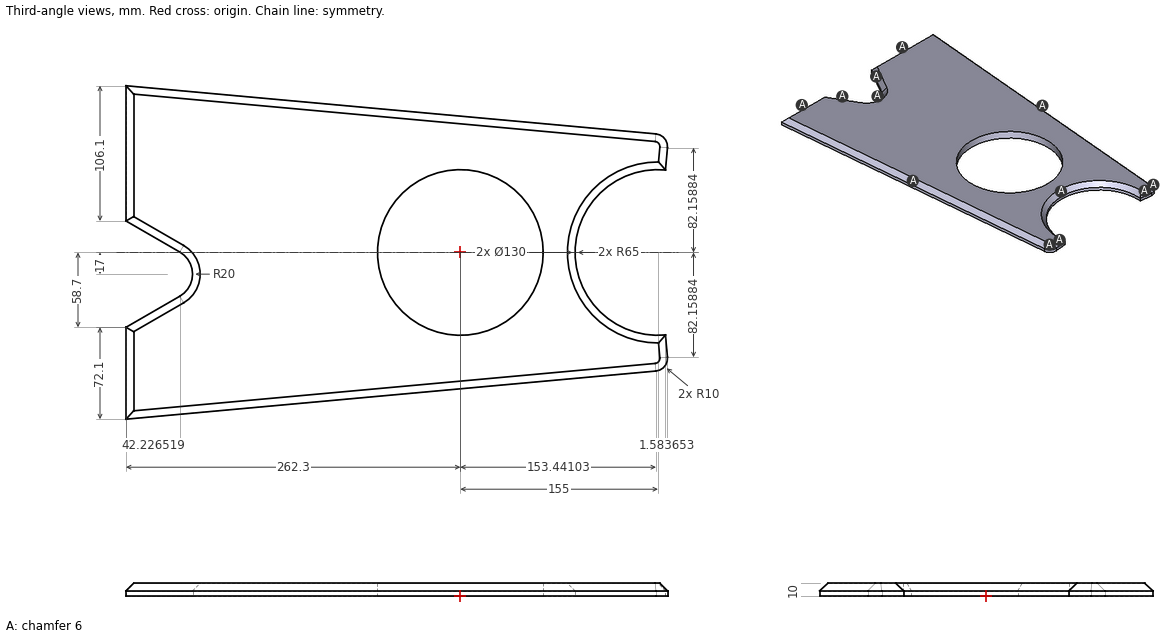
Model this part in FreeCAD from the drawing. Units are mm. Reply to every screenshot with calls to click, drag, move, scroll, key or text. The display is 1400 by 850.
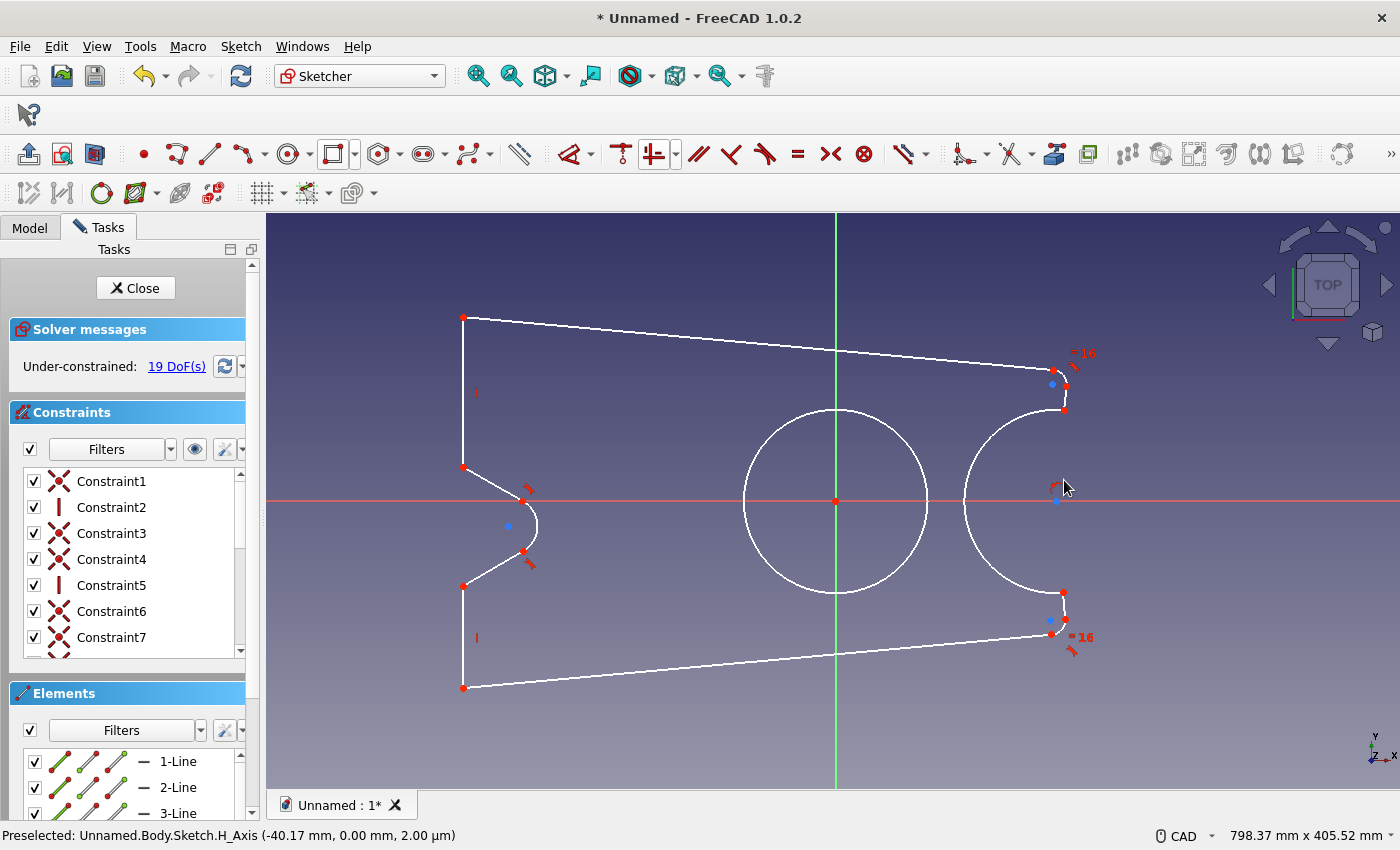
click(1051, 620)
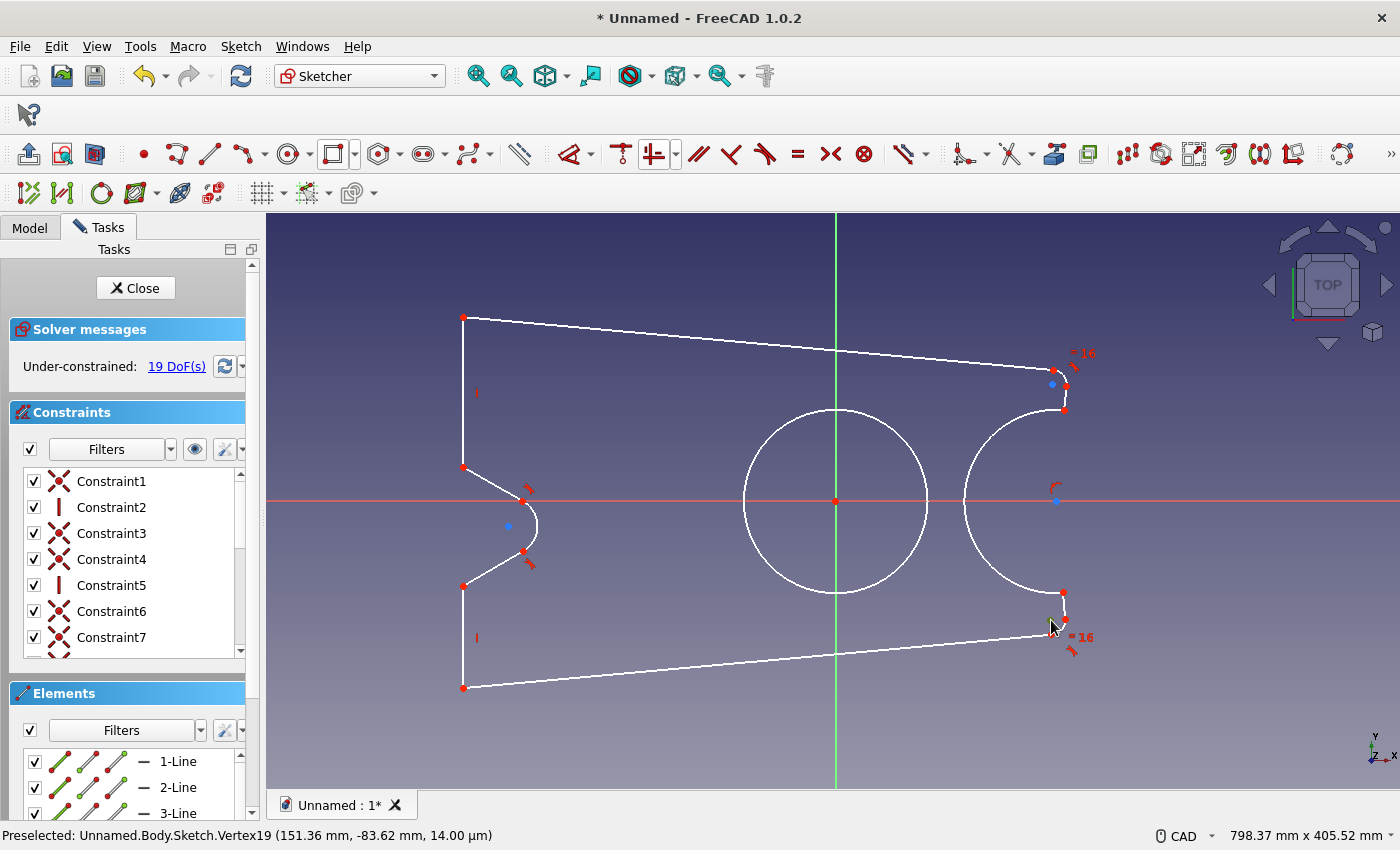
click(1052, 385)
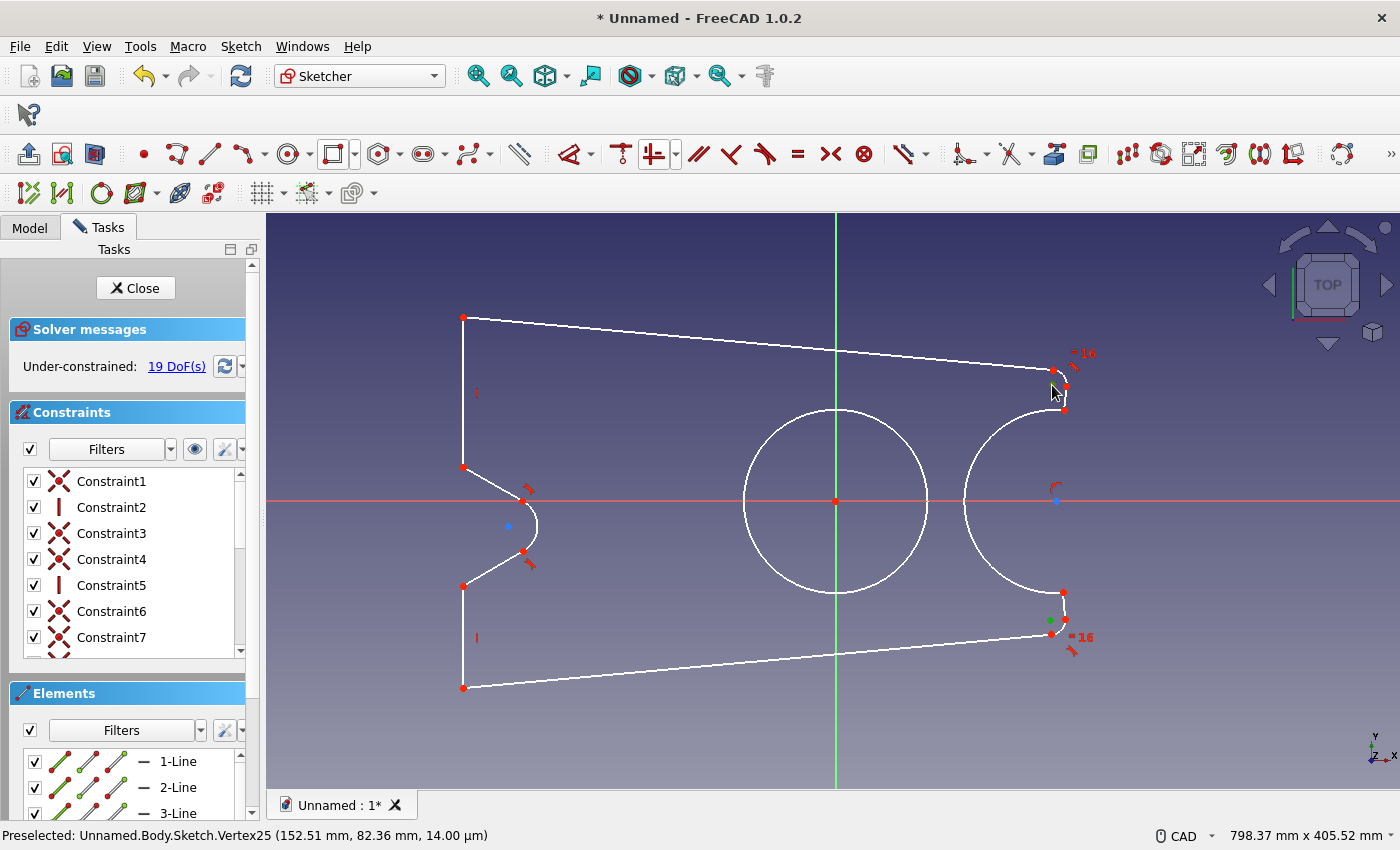
click(361, 501)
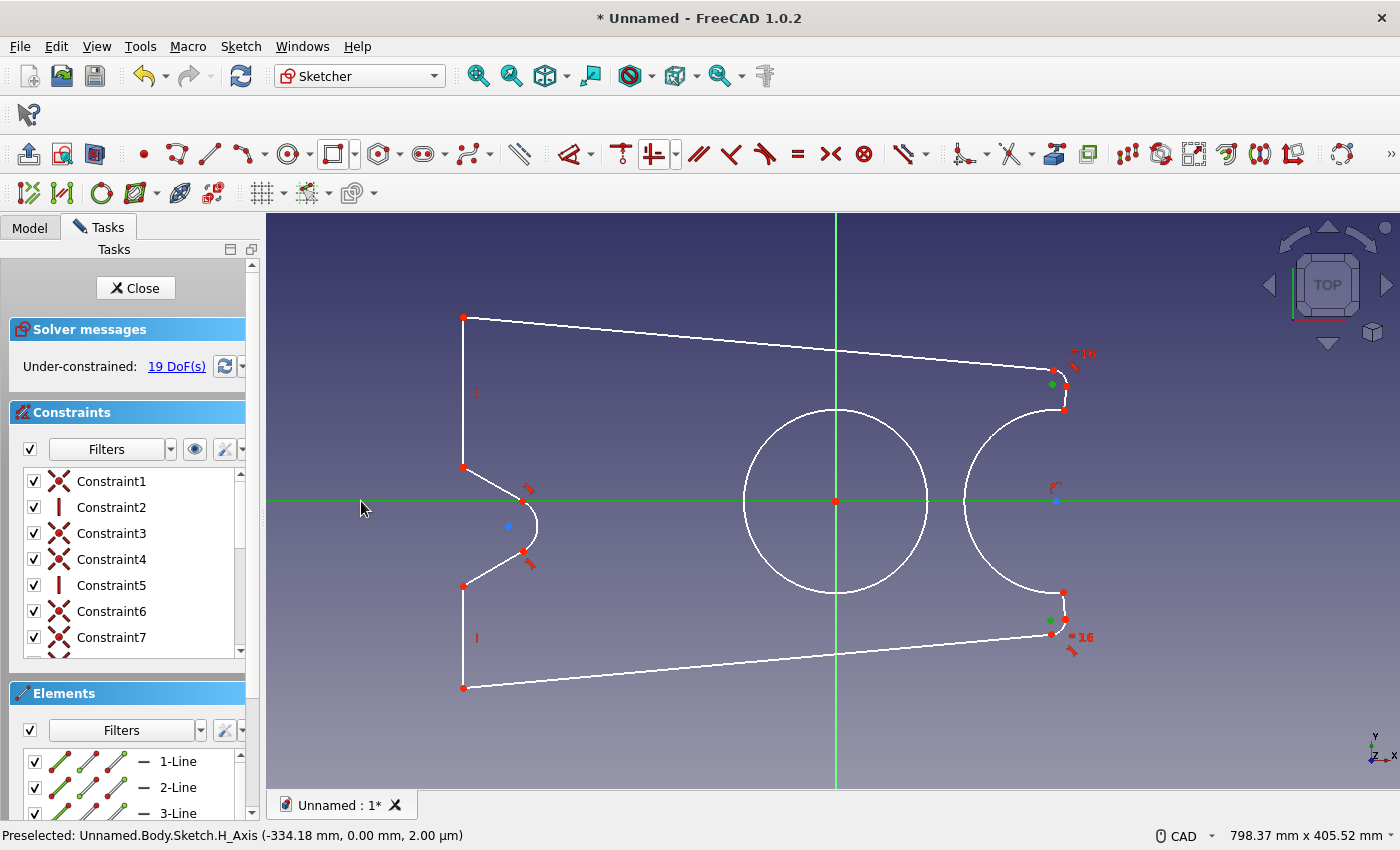
click(831, 154)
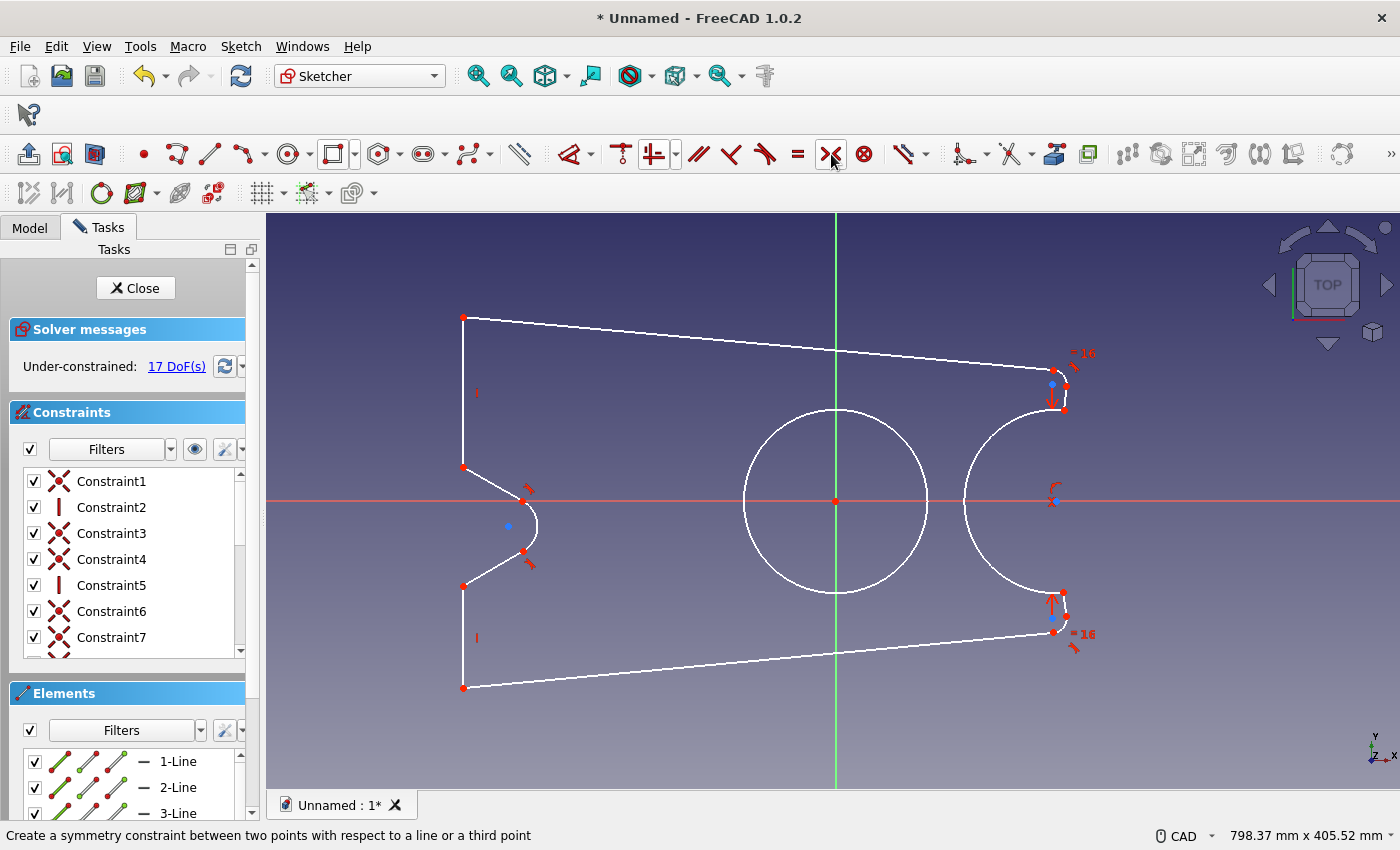
click(463, 688)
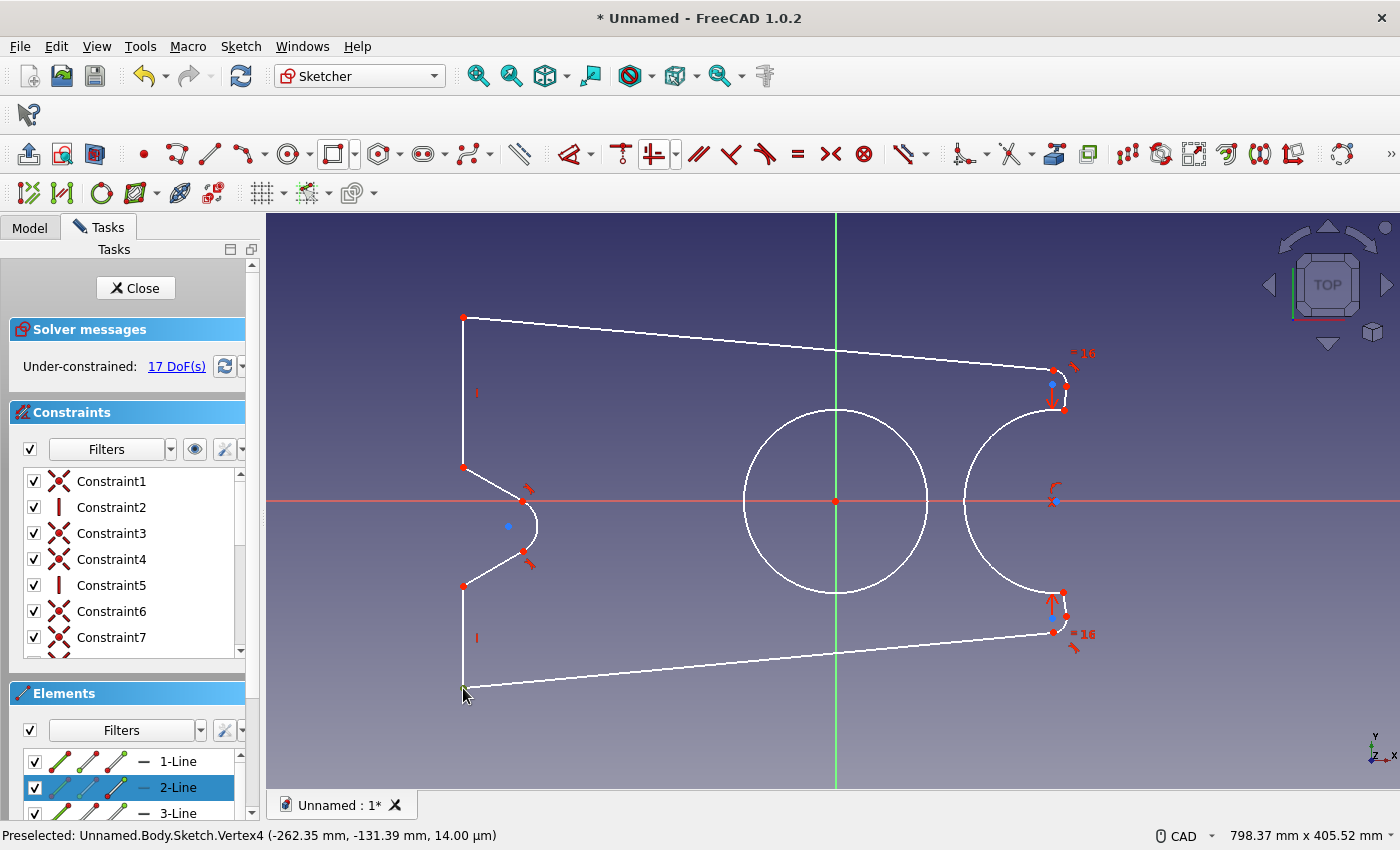
click(463, 317)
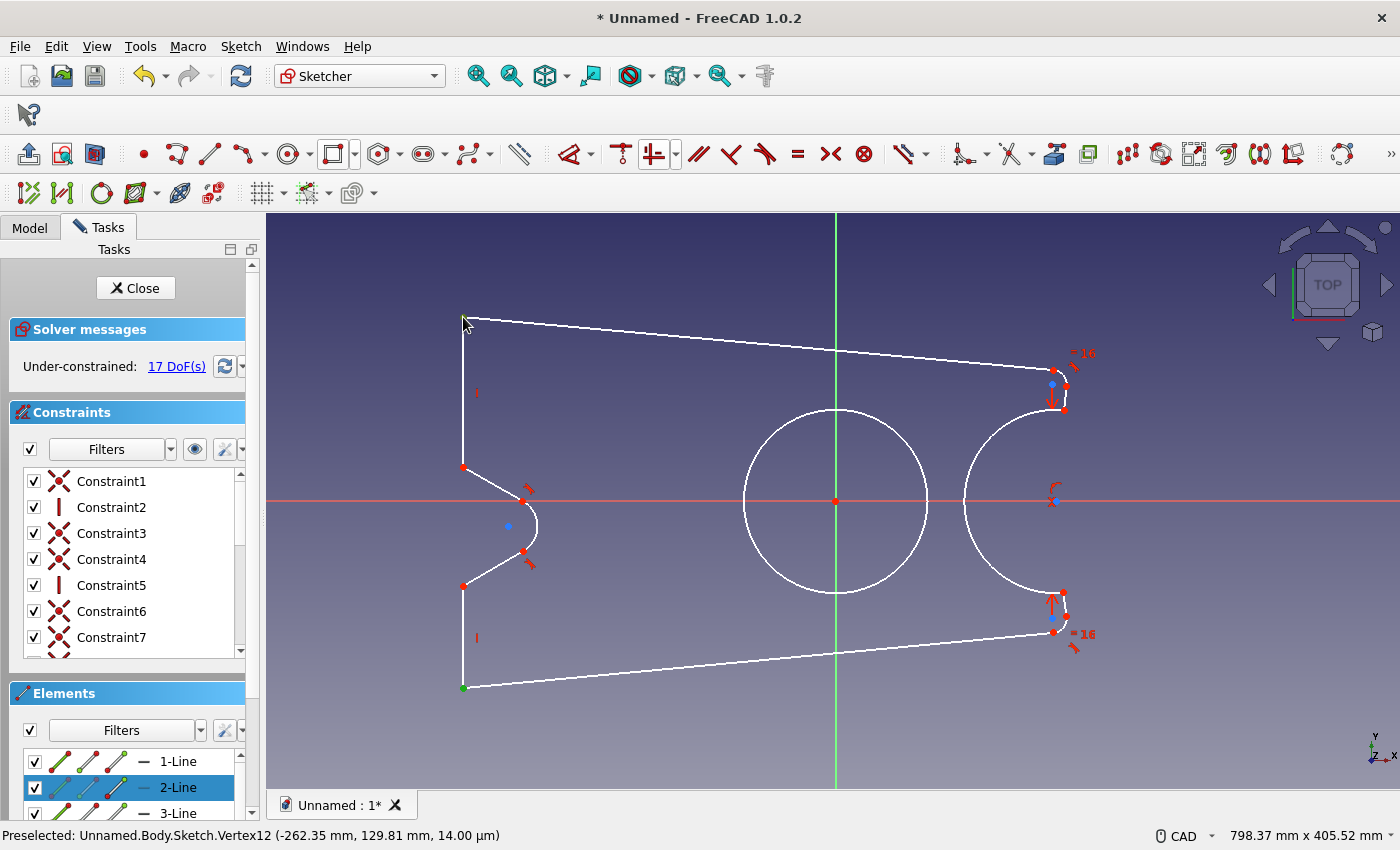
click(361, 501)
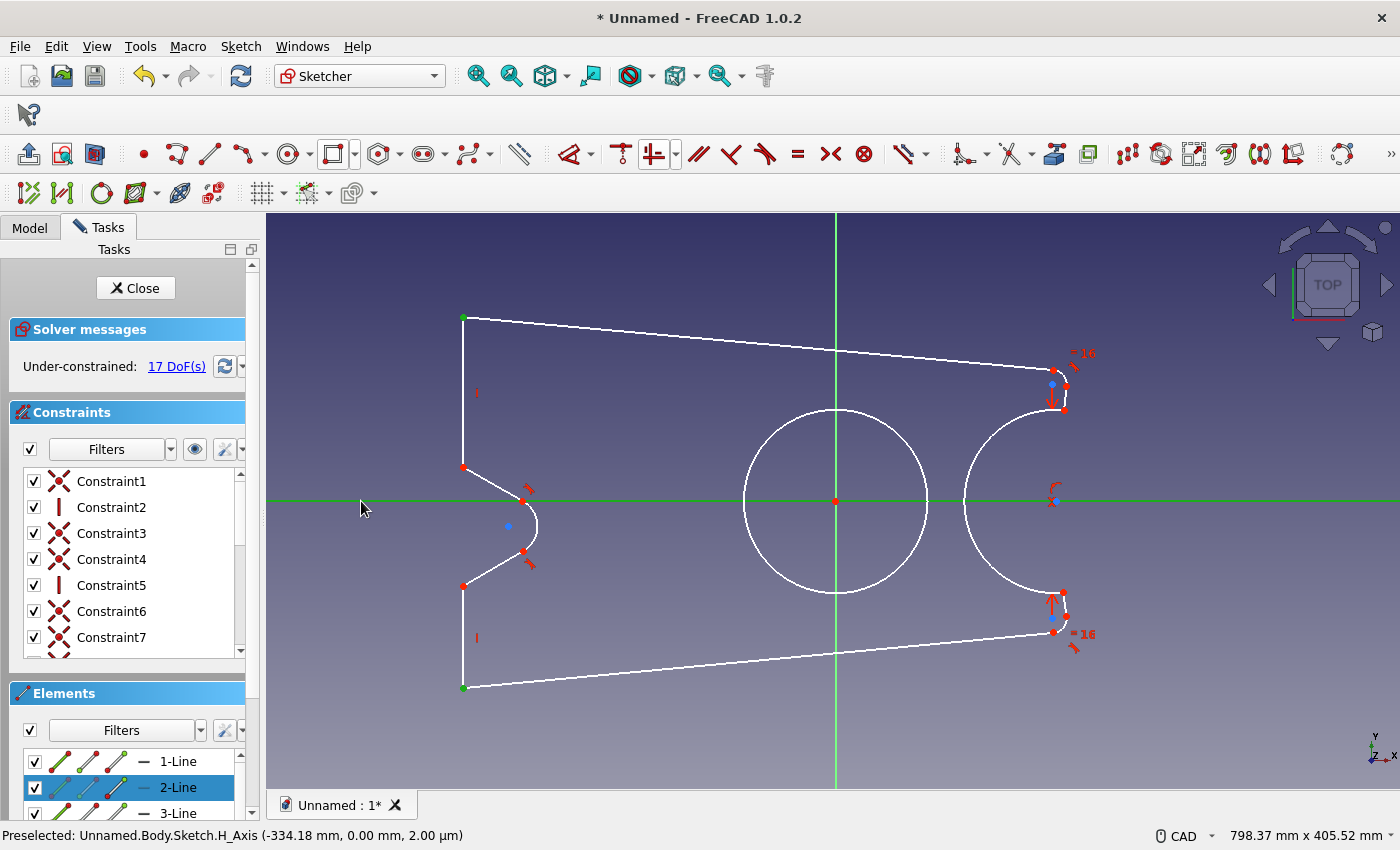
click(831, 154)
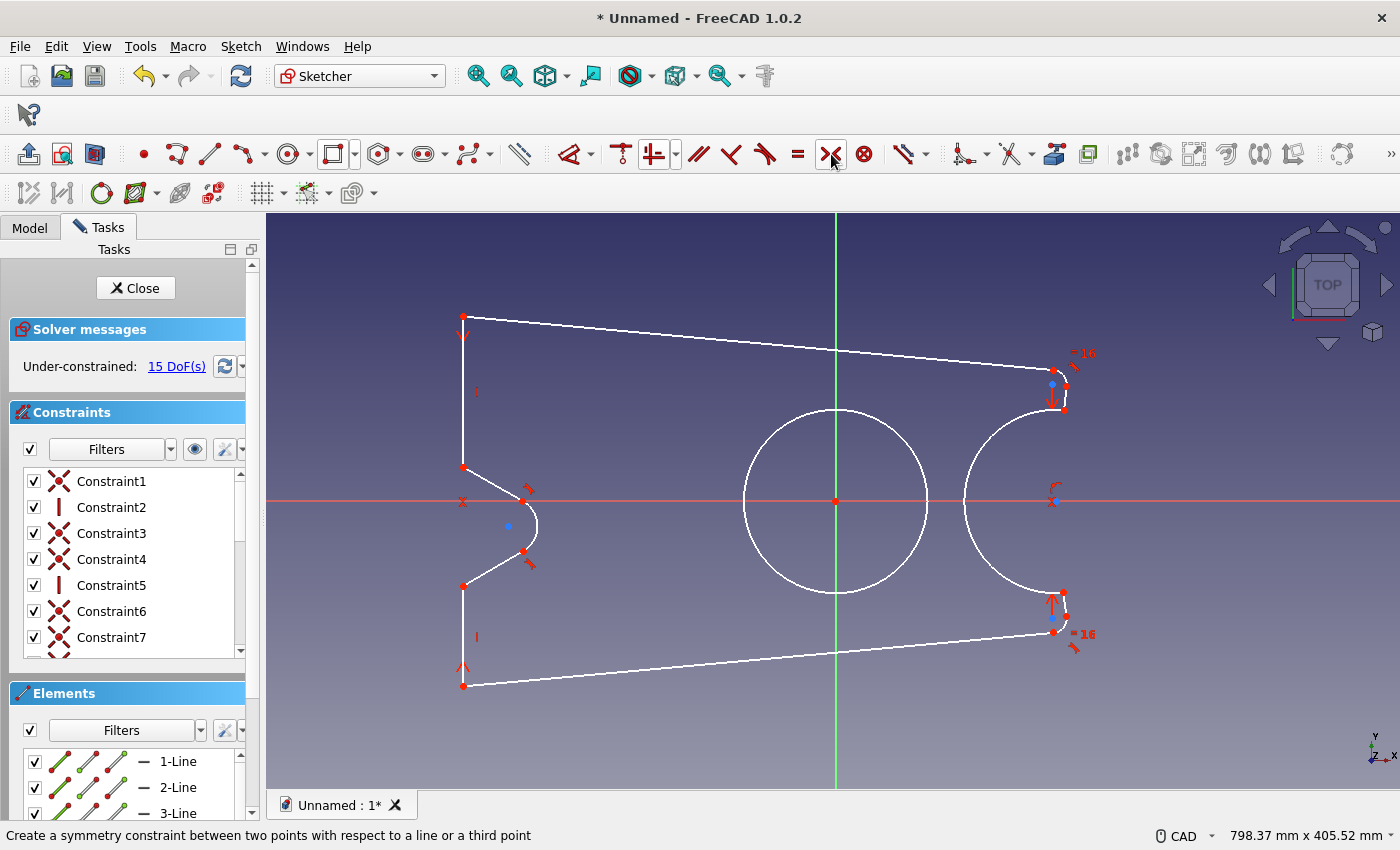
scroll(1064, 627, up, 6)